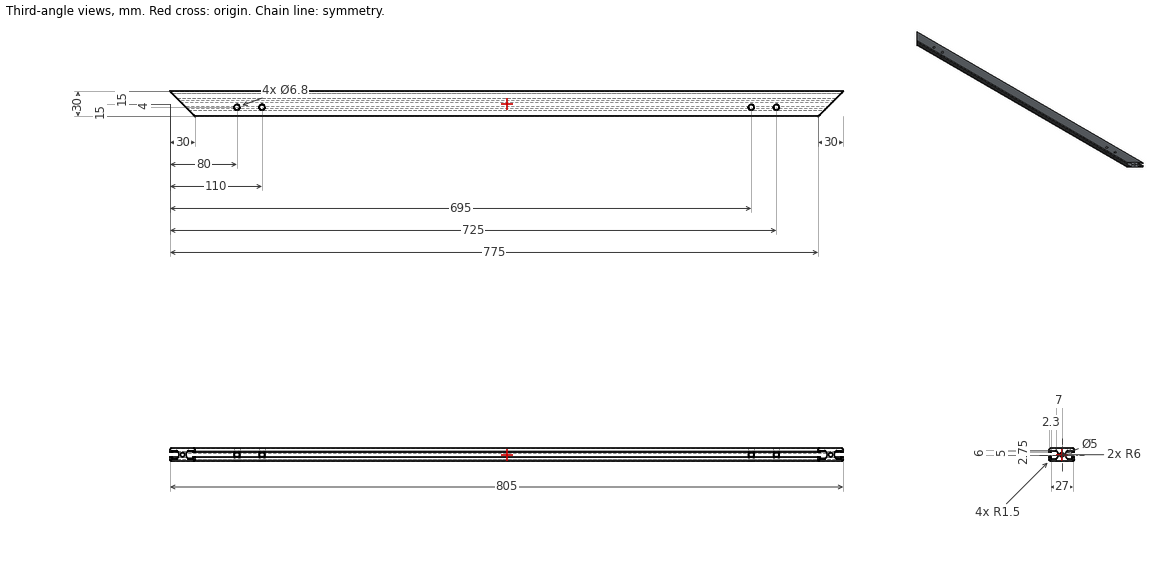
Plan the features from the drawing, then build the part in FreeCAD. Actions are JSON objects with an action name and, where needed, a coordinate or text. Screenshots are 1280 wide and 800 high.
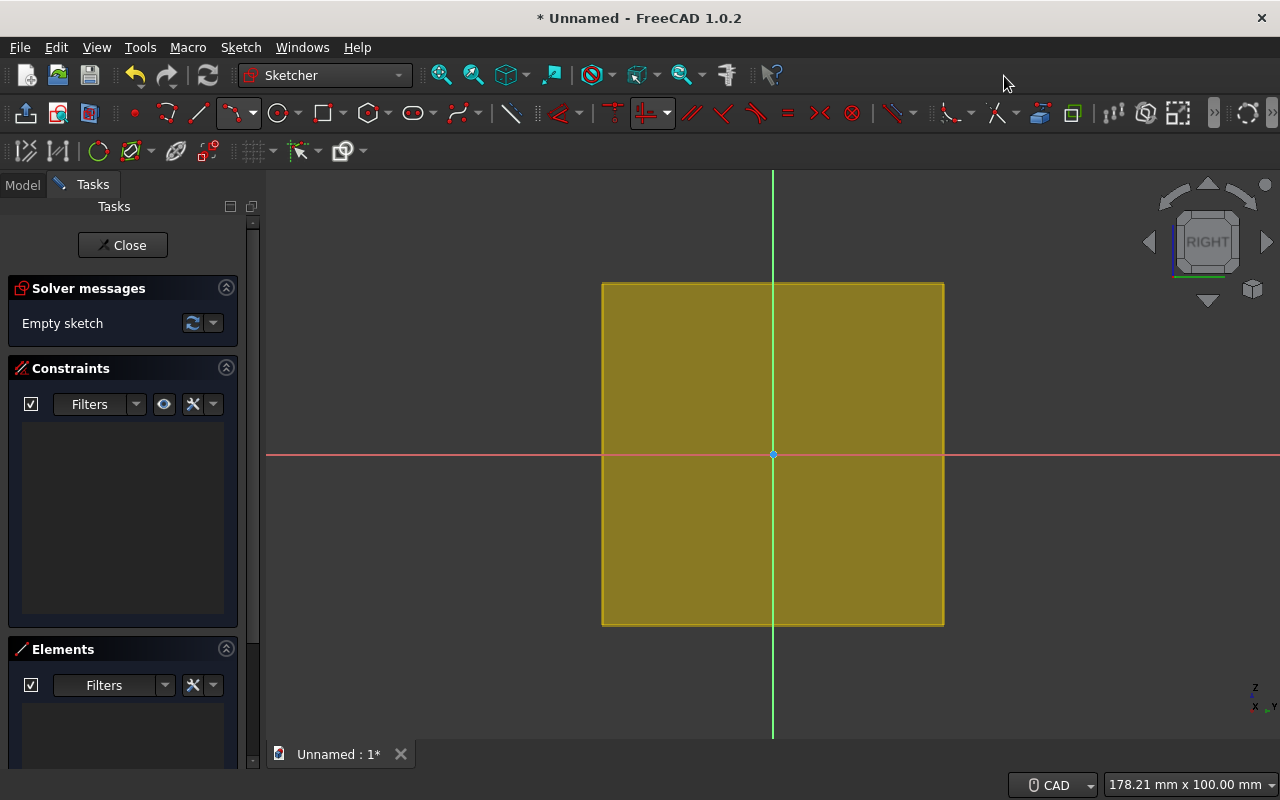
{"action": "scroll", "coordinate": [803, 455], "scroll_direction": "up", "scroll_amount": 6}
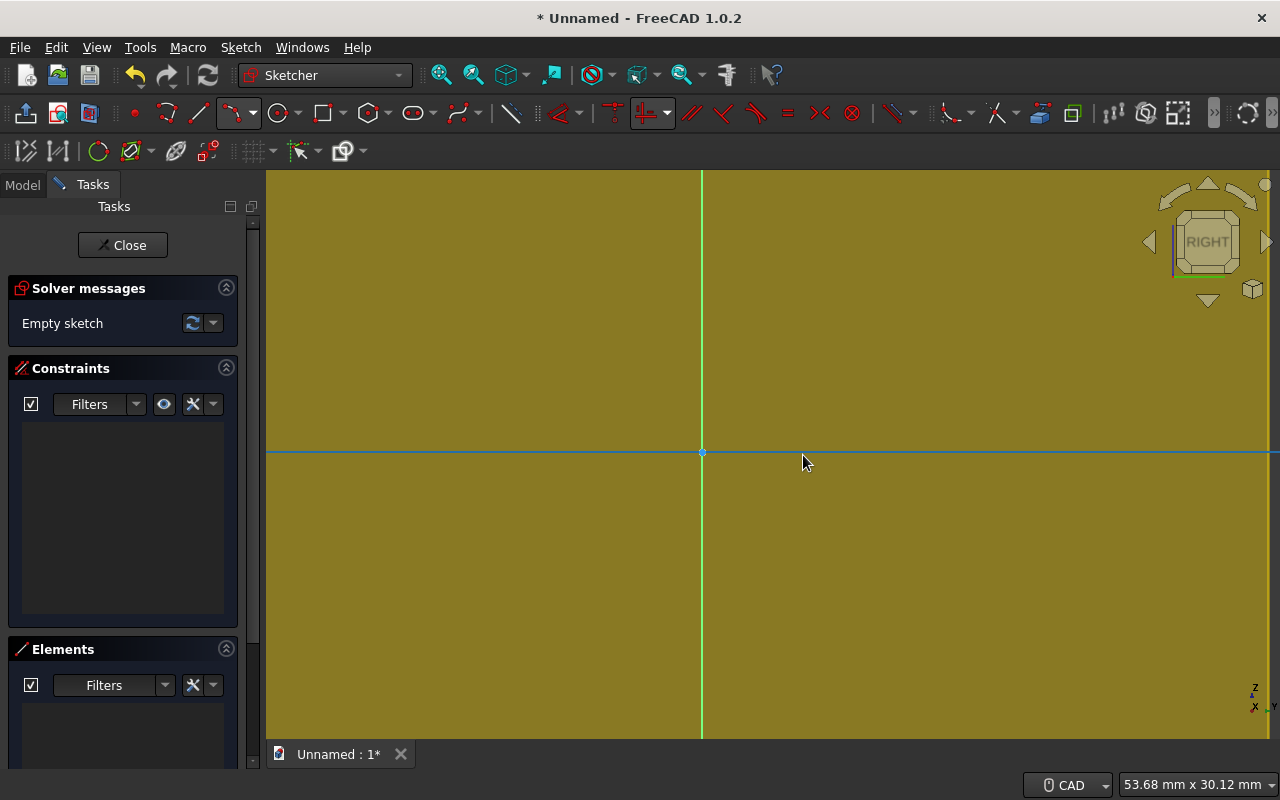
{"action": "left_click", "coordinate": [168, 114]}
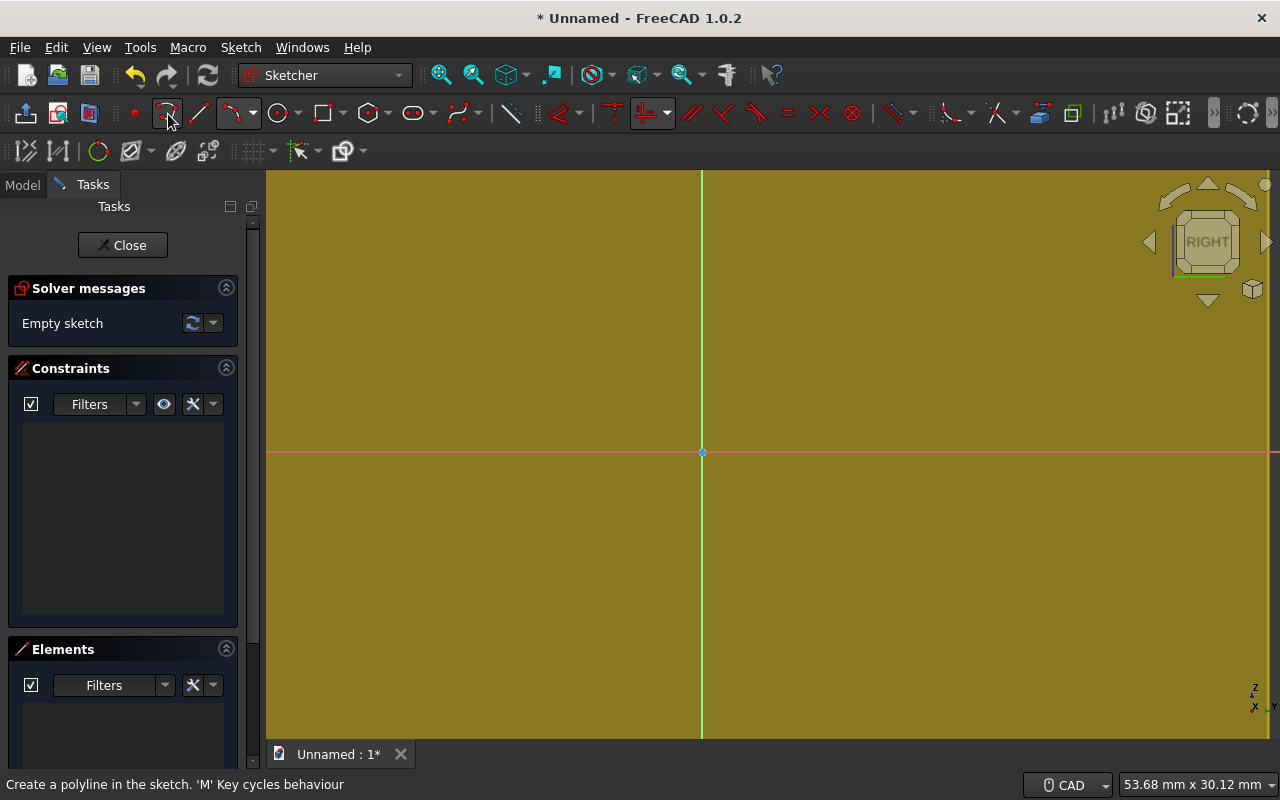
{"action": "left_click", "coordinate": [419, 339]}
{"action": "left_click", "coordinate": [419, 391]}
{"action": "left_click", "coordinate": [462, 391]}
{"action": "left_click", "coordinate": [462, 358]}
{"action": "left_click", "coordinate": [570, 358]}
{"action": "right_click", "coordinate": [570, 358]}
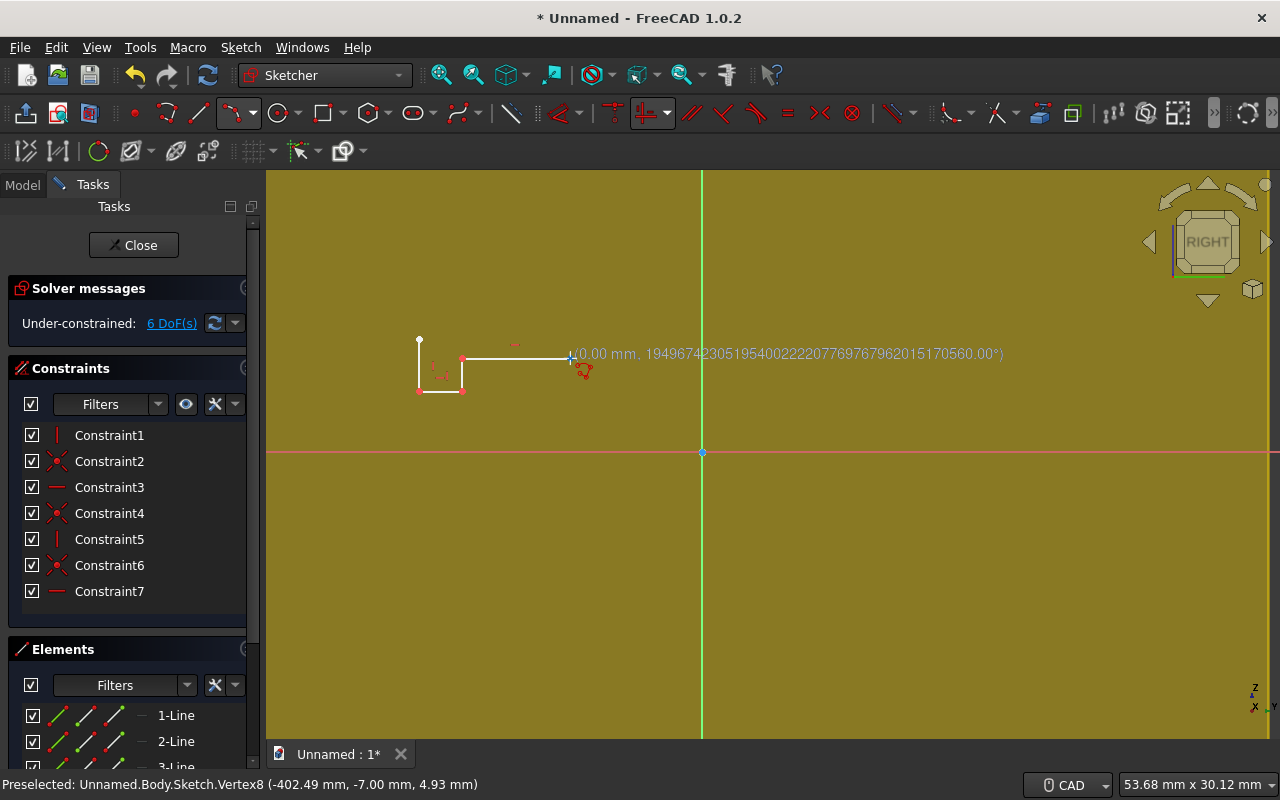
{"action": "left_click", "coordinate": [570, 547]}
{"action": "left_click", "coordinate": [462, 547]}
{"action": "left_click", "coordinate": [462, 514]}
{"action": "left_click", "coordinate": [419, 514]}
{"action": "left_click", "coordinate": [419, 566]}
{"action": "right_click", "coordinate": [419, 566]}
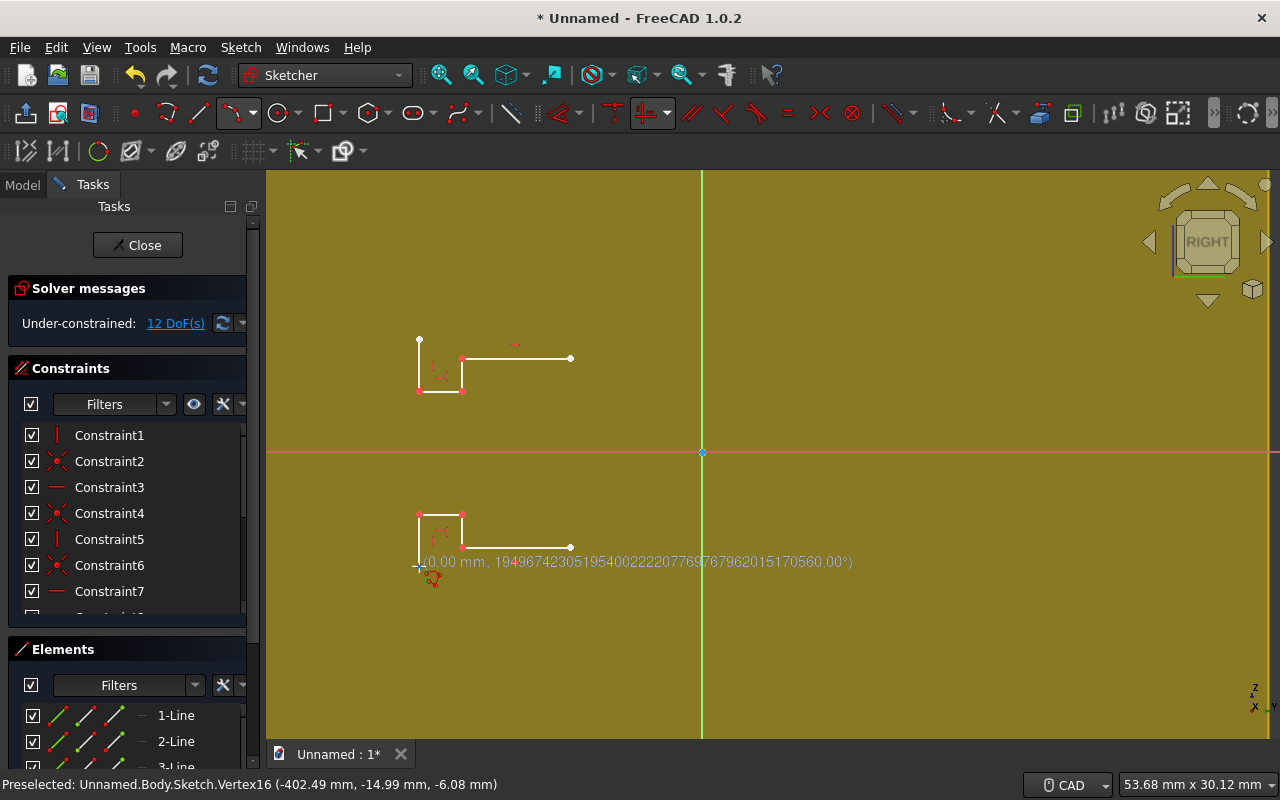
{"action": "left_click", "coordinate": [200, 114]}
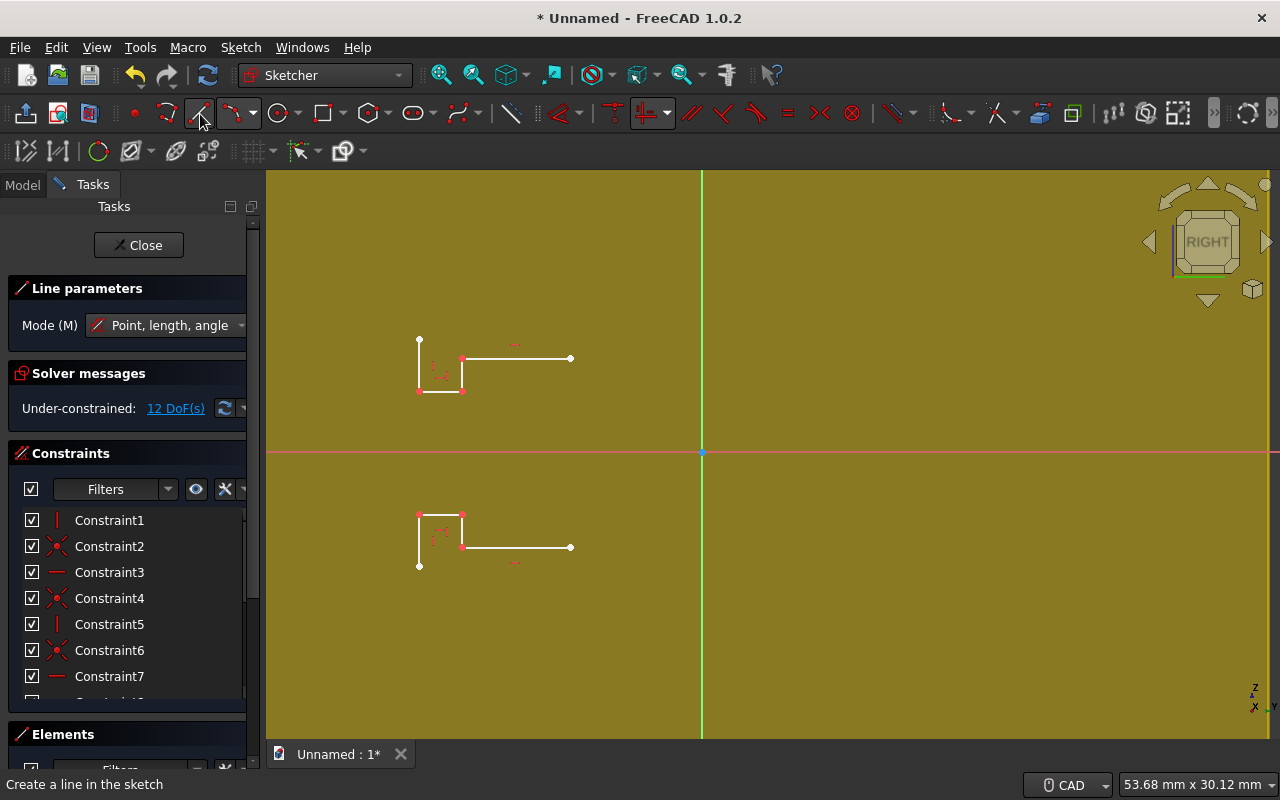
{"action": "left_click", "coordinate": [447, 594]}
{"action": "left_click", "coordinate": [957, 594]}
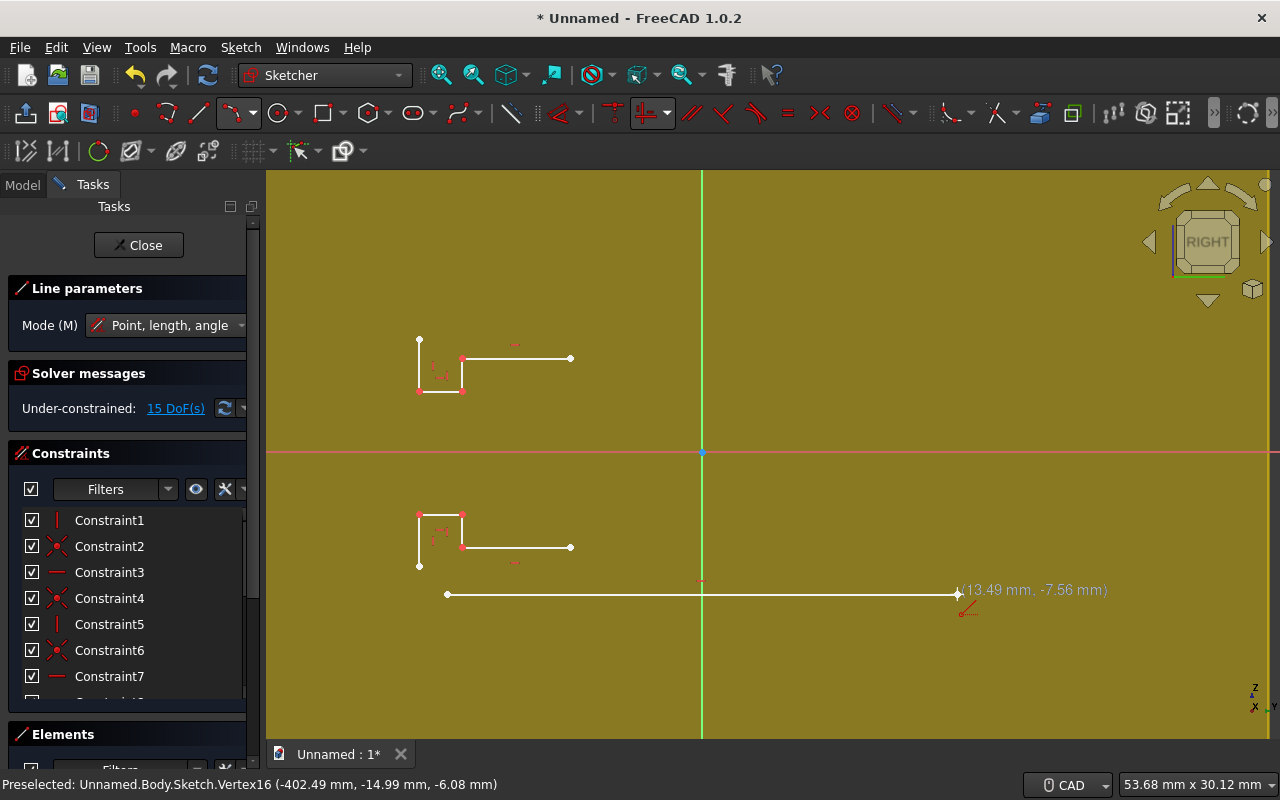
{"action": "left_click", "coordinate": [168, 114]}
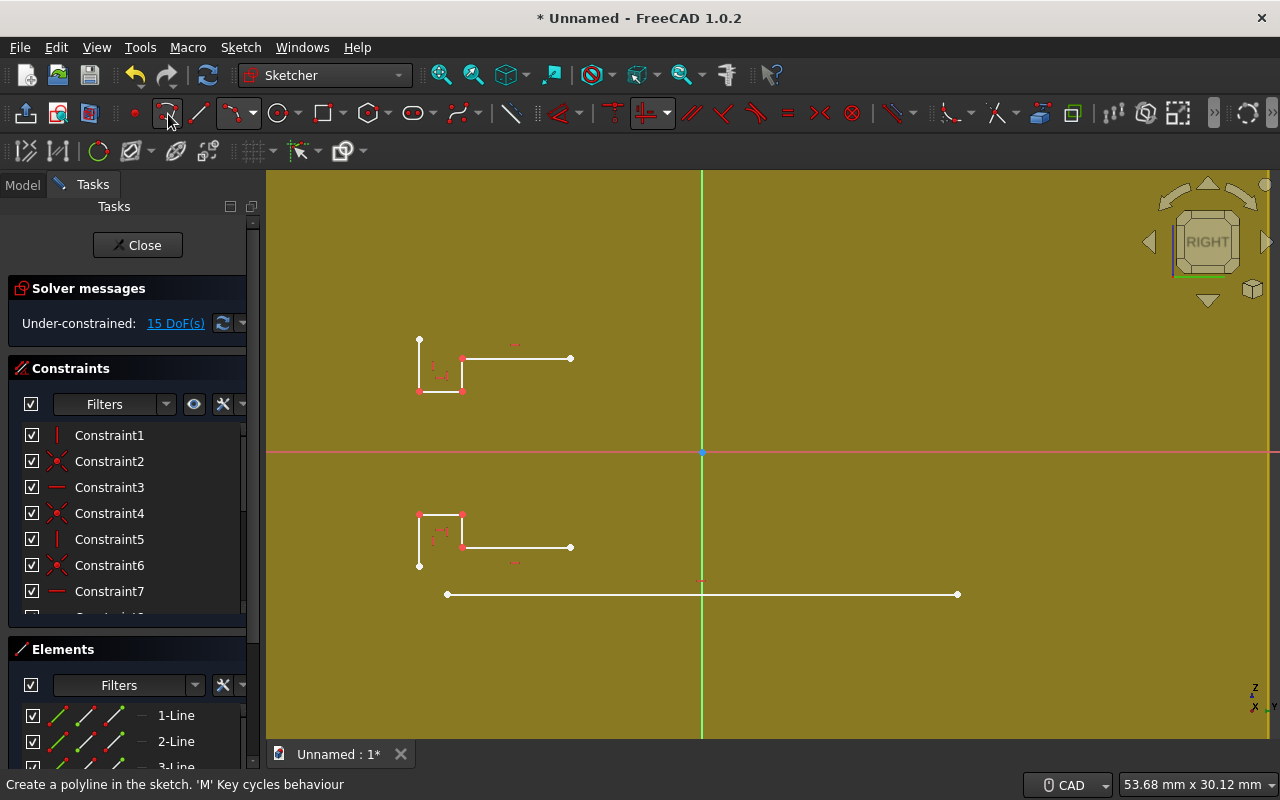
{"action": "left_click", "coordinate": [986, 566]}
{"action": "left_click", "coordinate": [986, 514]}
{"action": "left_click", "coordinate": [942, 514]}
{"action": "left_click", "coordinate": [942, 547]}
{"action": "left_click", "coordinate": [834, 547]}
{"action": "right_click", "coordinate": [834, 547]}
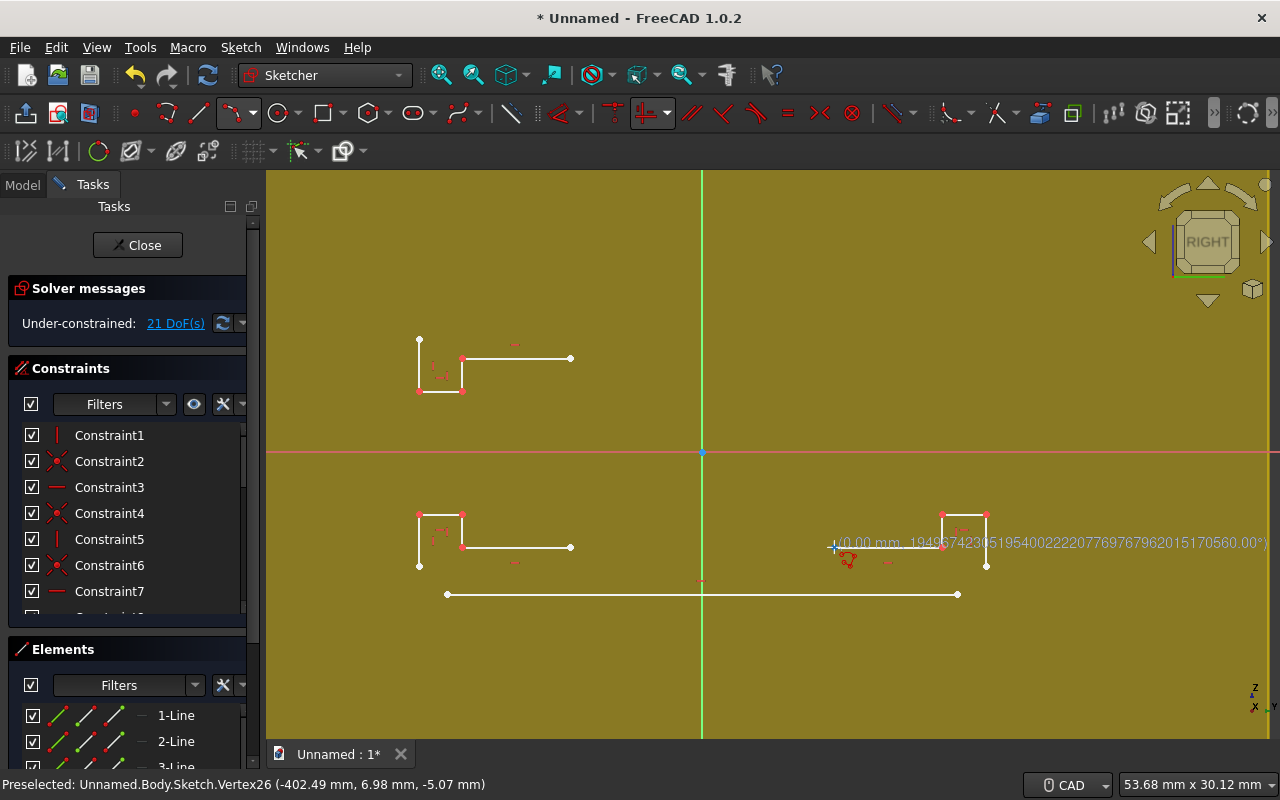
{"action": "left_click", "coordinate": [834, 358]}
{"action": "left_click", "coordinate": [942, 358]}
{"action": "left_click", "coordinate": [942, 391]}
{"action": "left_click", "coordinate": [986, 391]}
{"action": "left_click", "coordinate": [986, 339]}
{"action": "right_click", "coordinate": [986, 339]}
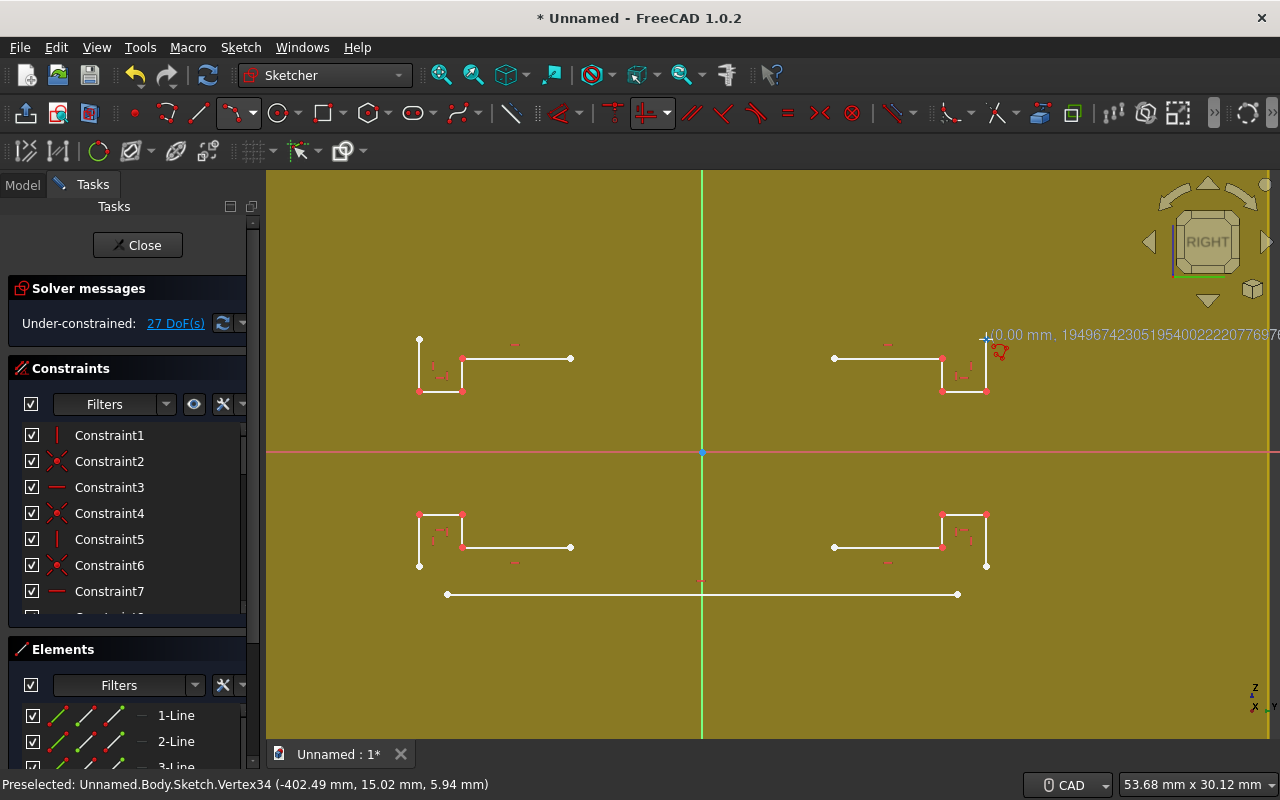
{"action": "left_click", "coordinate": [200, 114]}